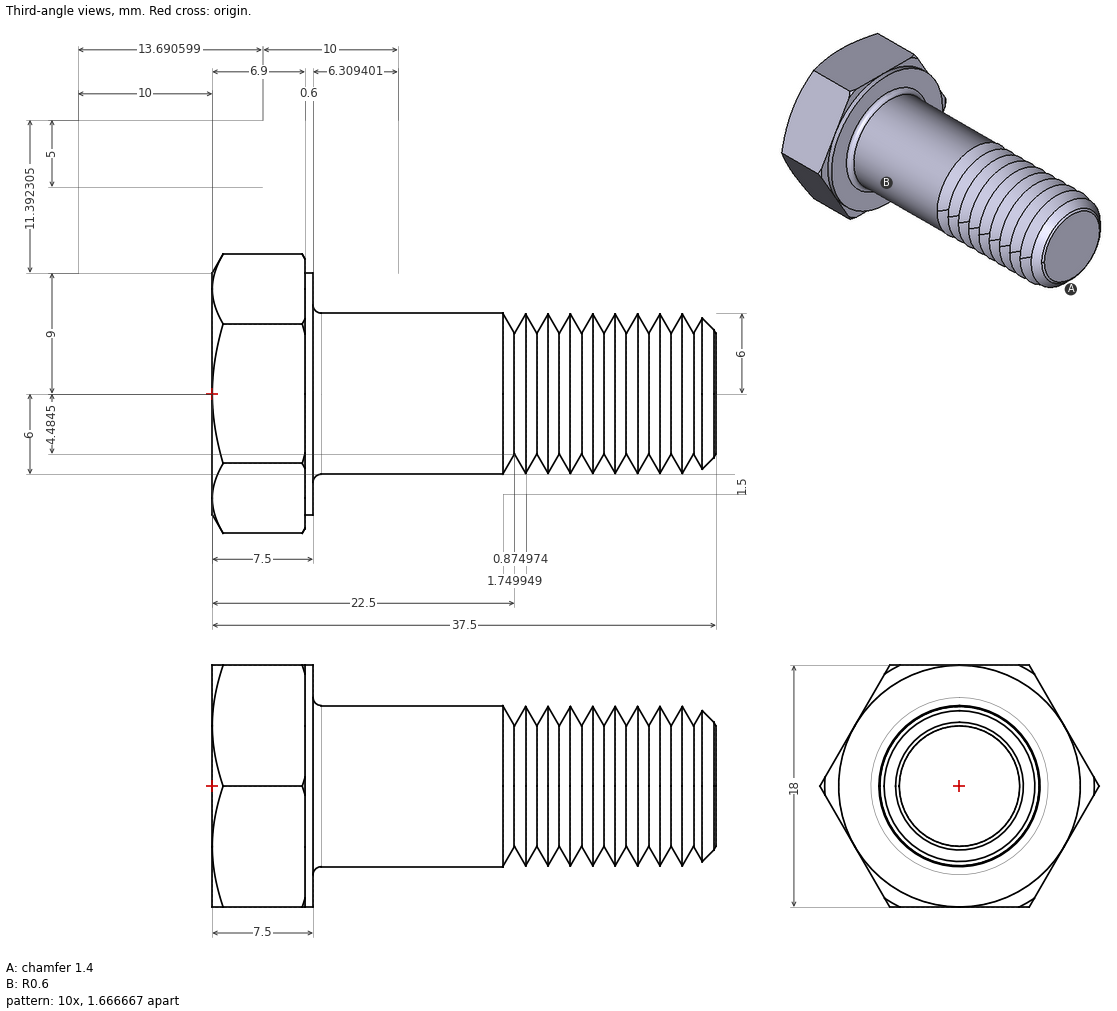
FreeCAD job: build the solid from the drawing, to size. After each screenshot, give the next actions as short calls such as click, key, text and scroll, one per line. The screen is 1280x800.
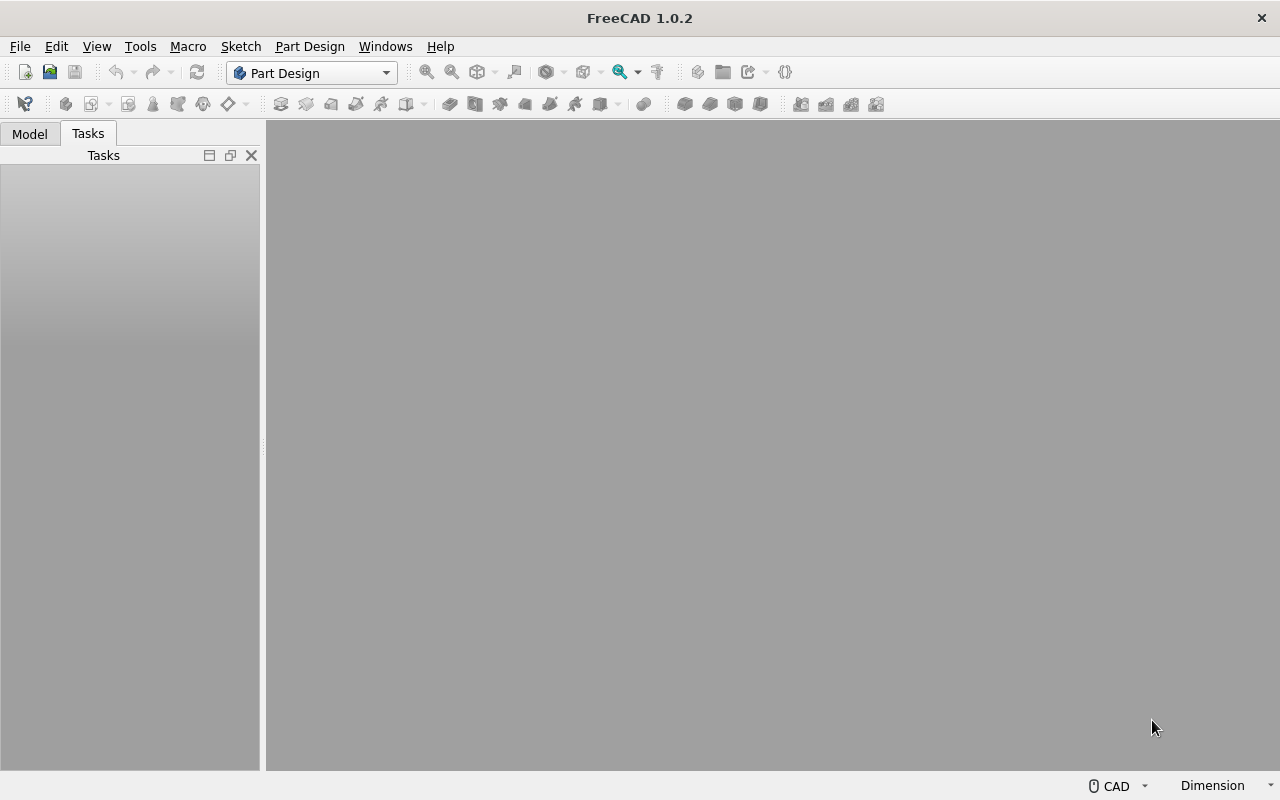
click(25, 72)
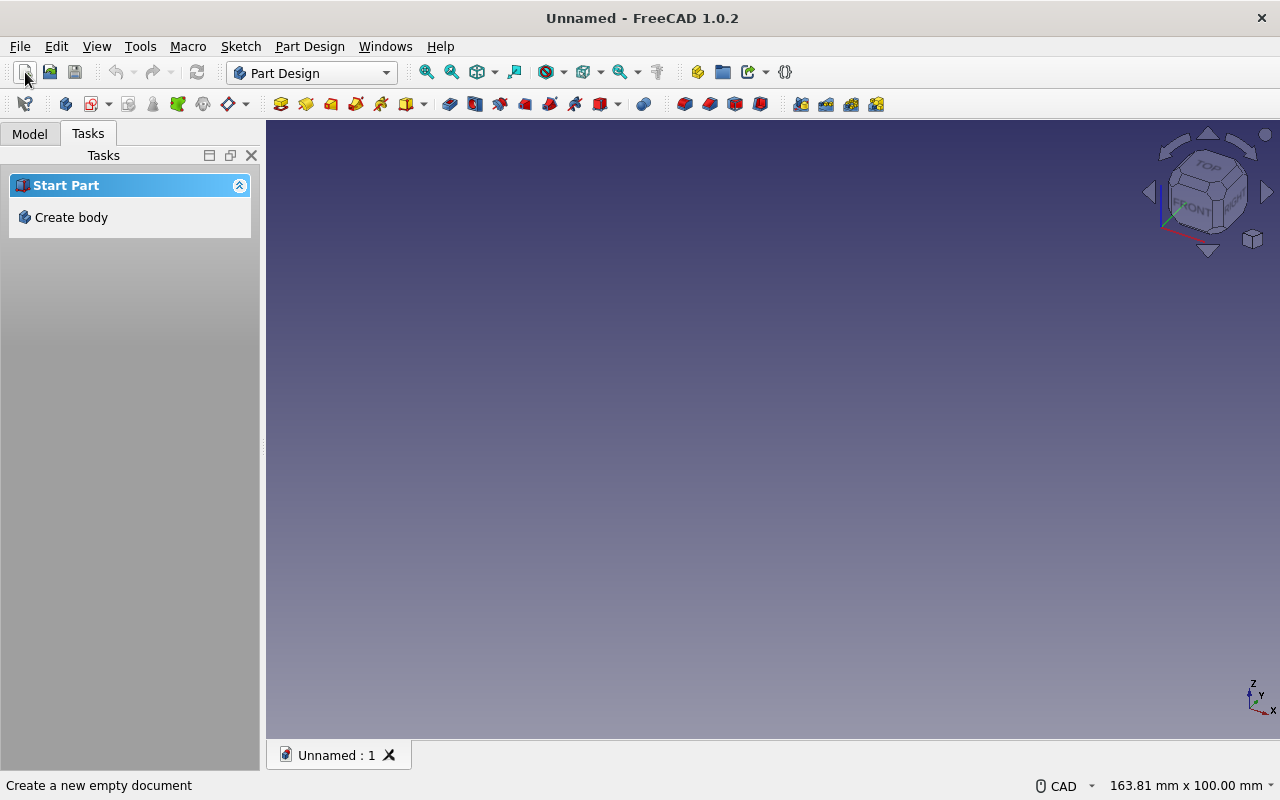
click(90, 104)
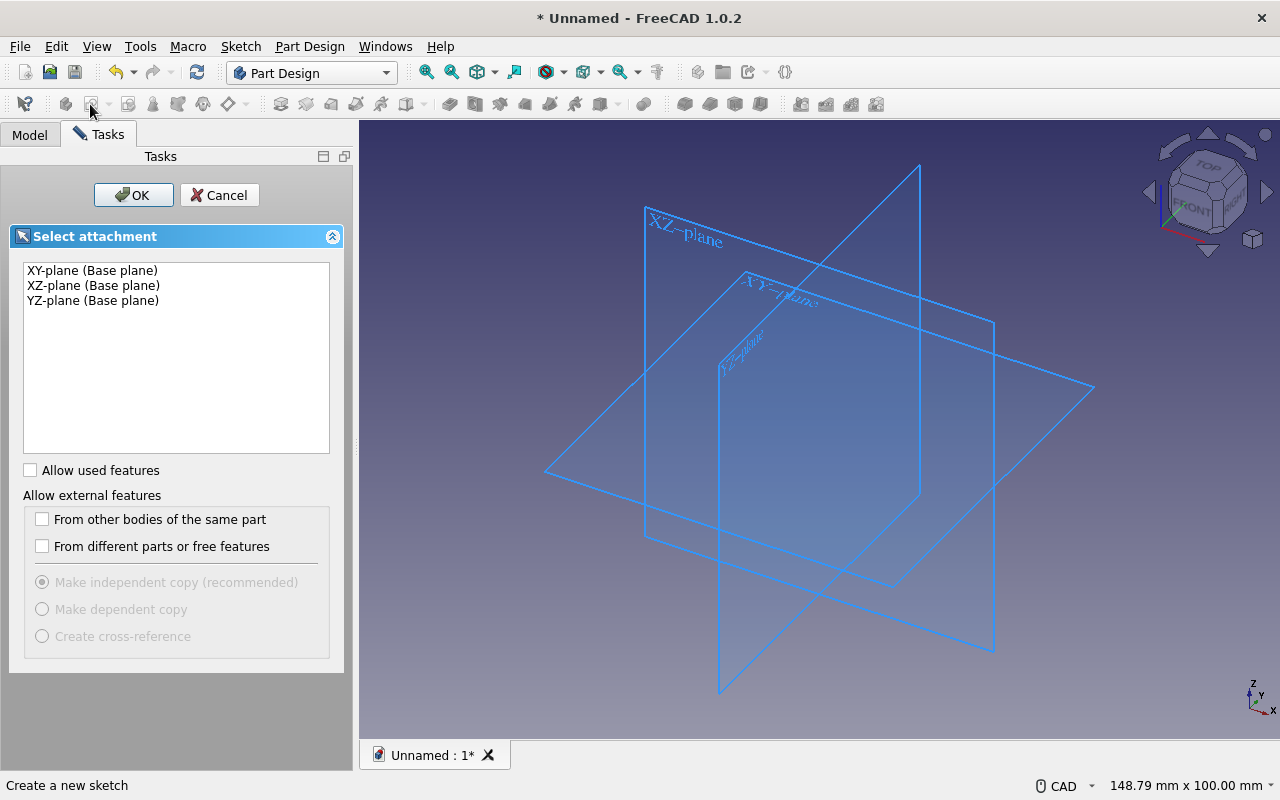
click(84, 300)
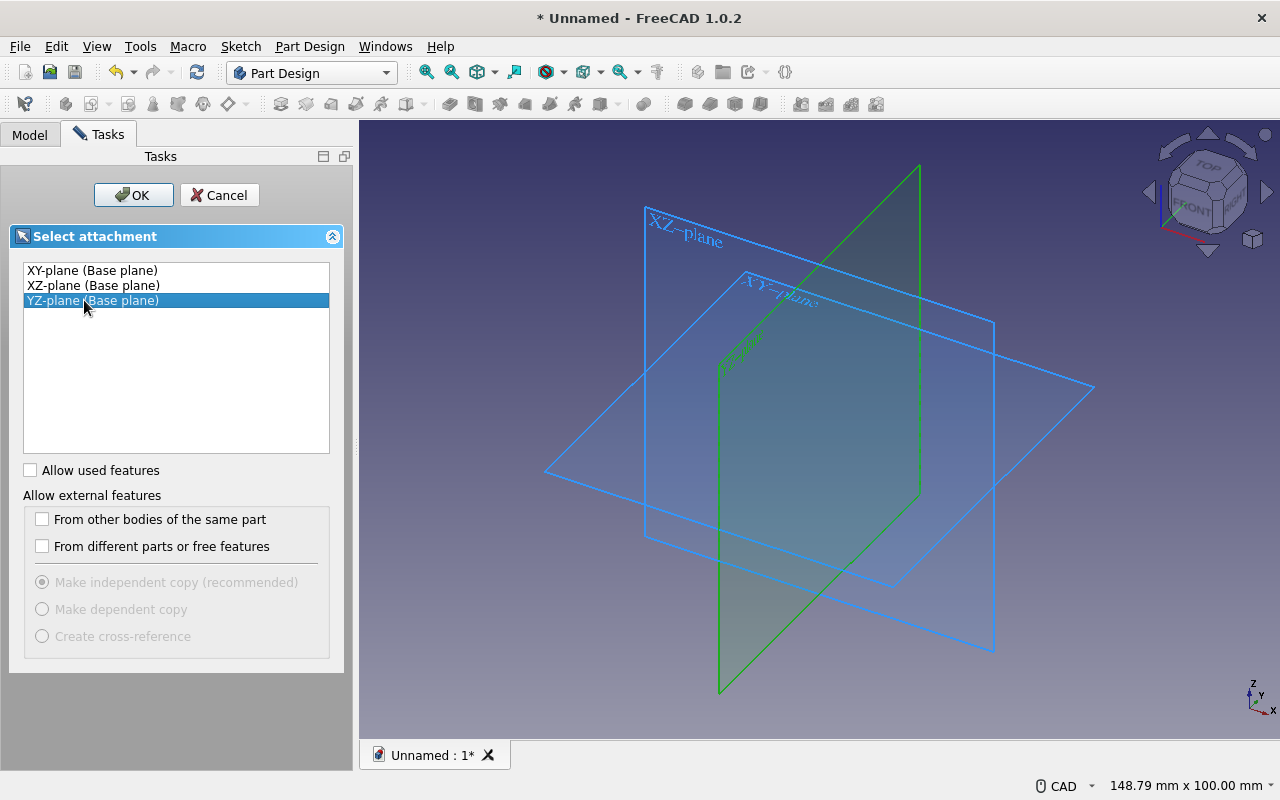
click(134, 195)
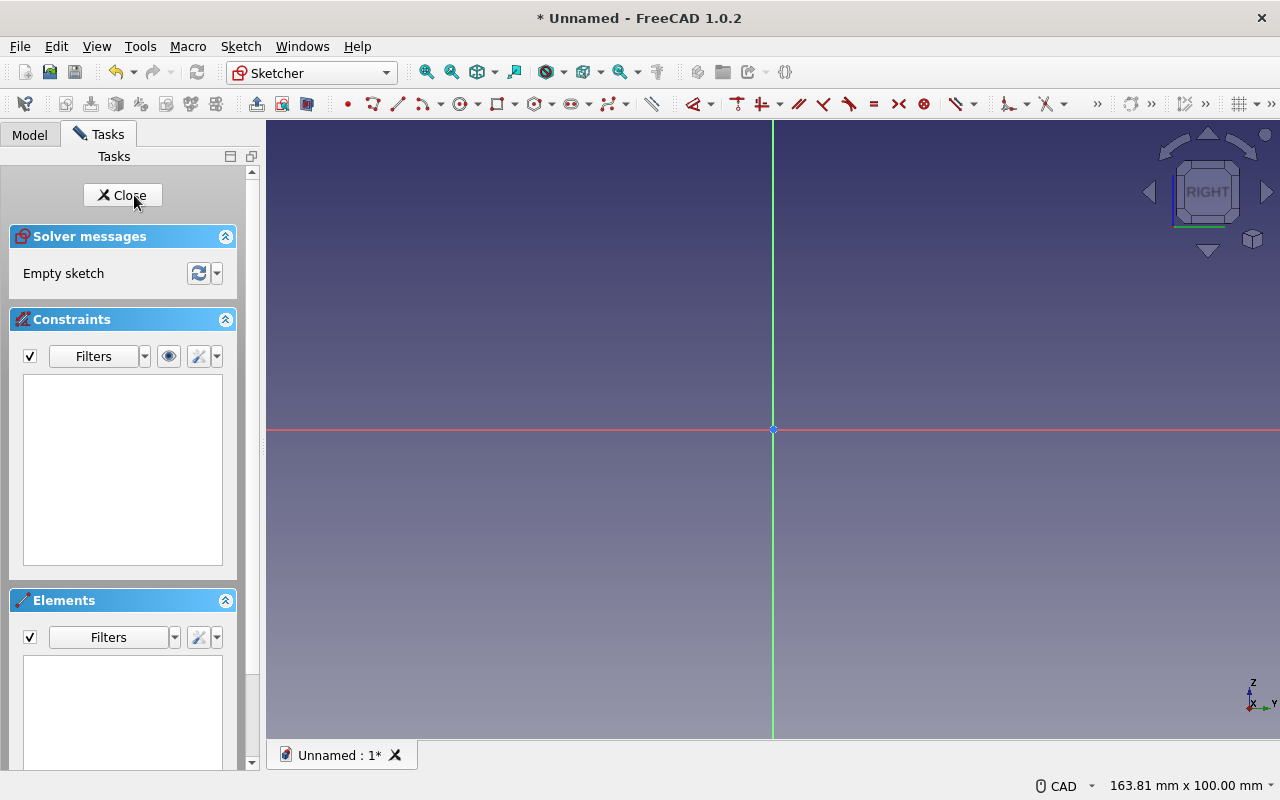
scroll(803, 430, up, 6)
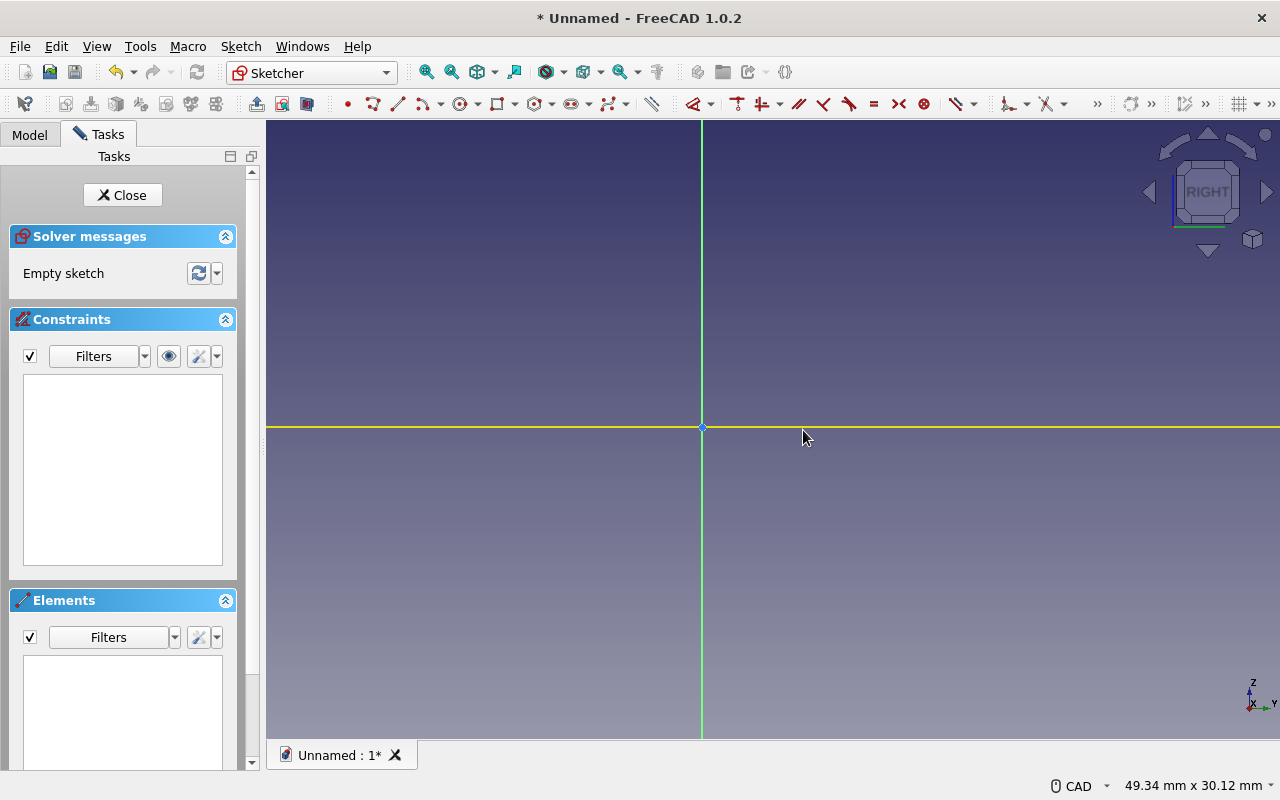
click(534, 104)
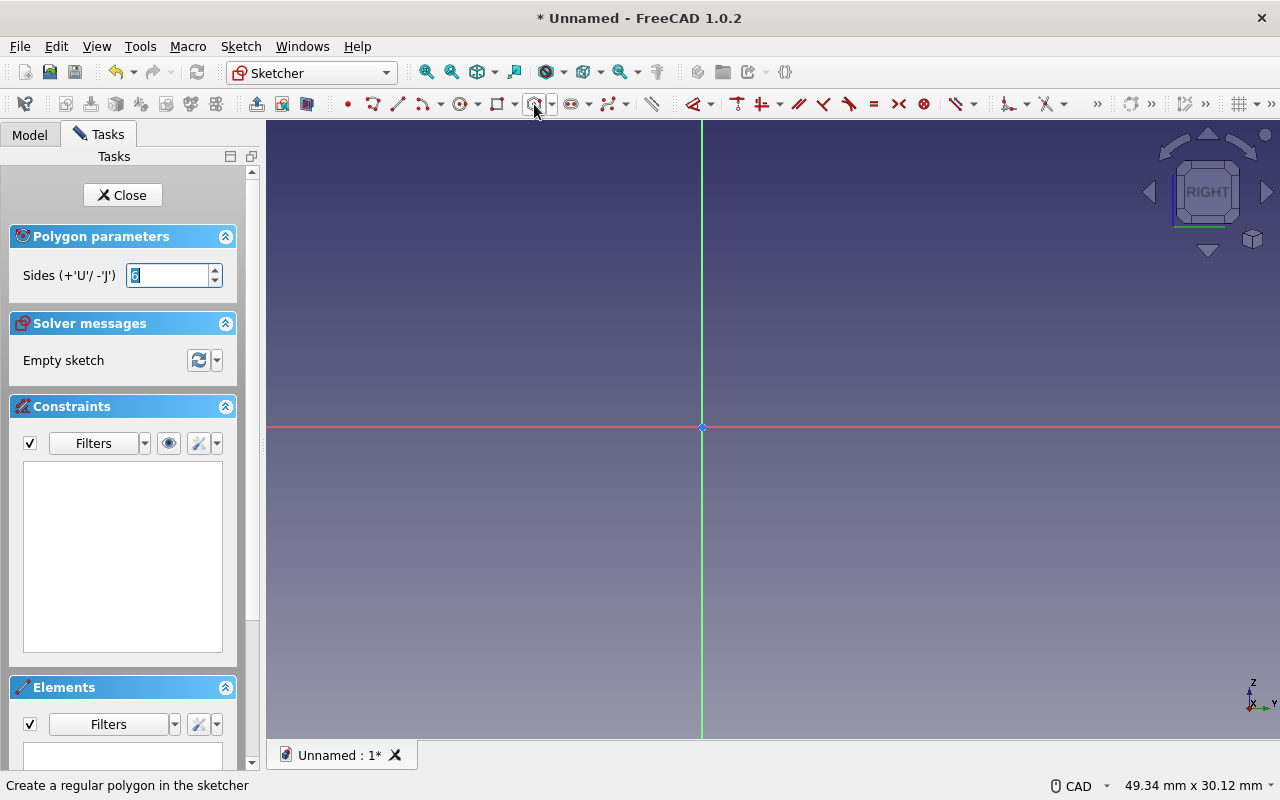
click(702, 427)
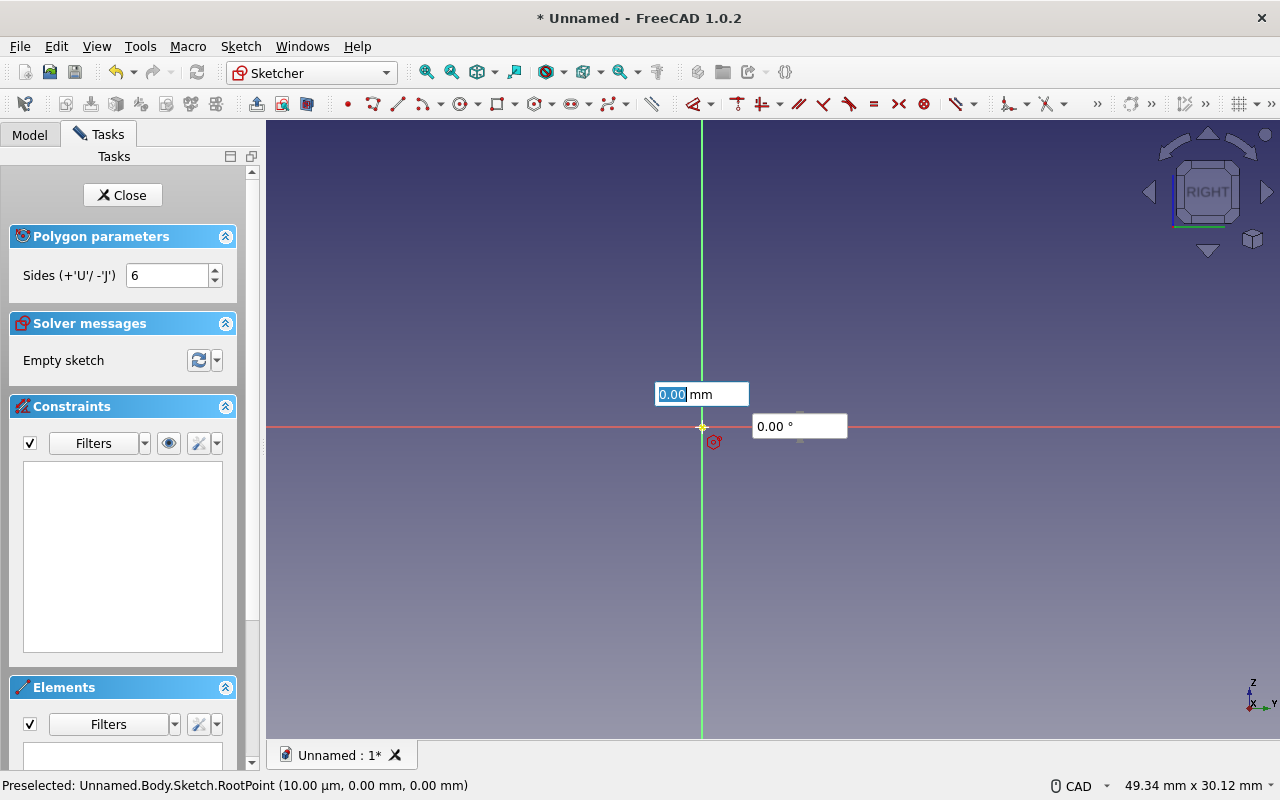
click(916, 427)
key(Escape)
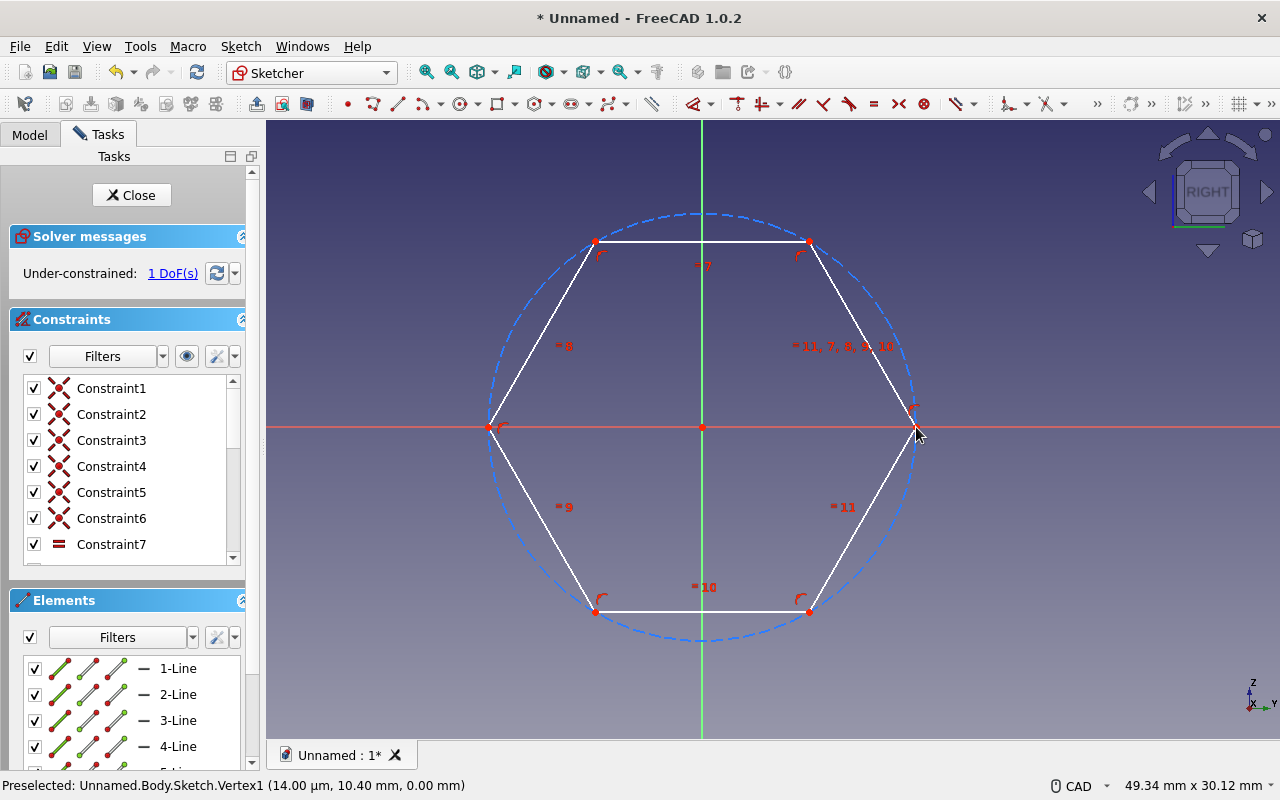
click(595, 612)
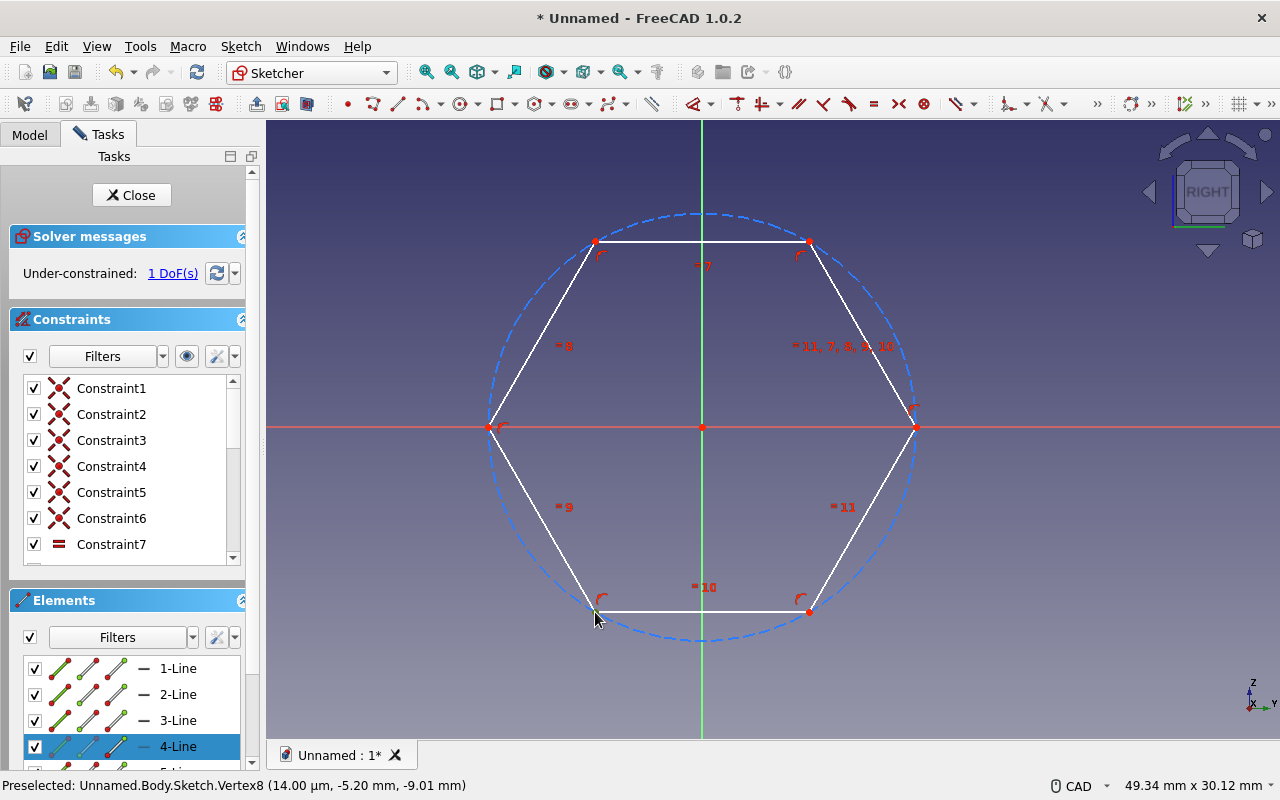
click(809, 242)